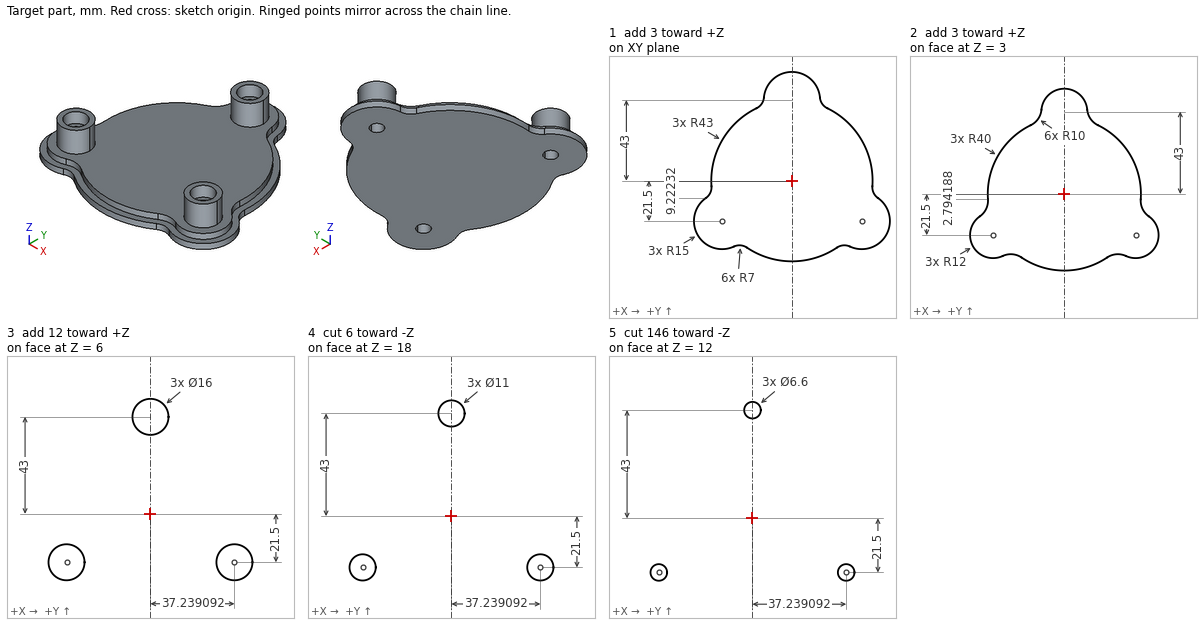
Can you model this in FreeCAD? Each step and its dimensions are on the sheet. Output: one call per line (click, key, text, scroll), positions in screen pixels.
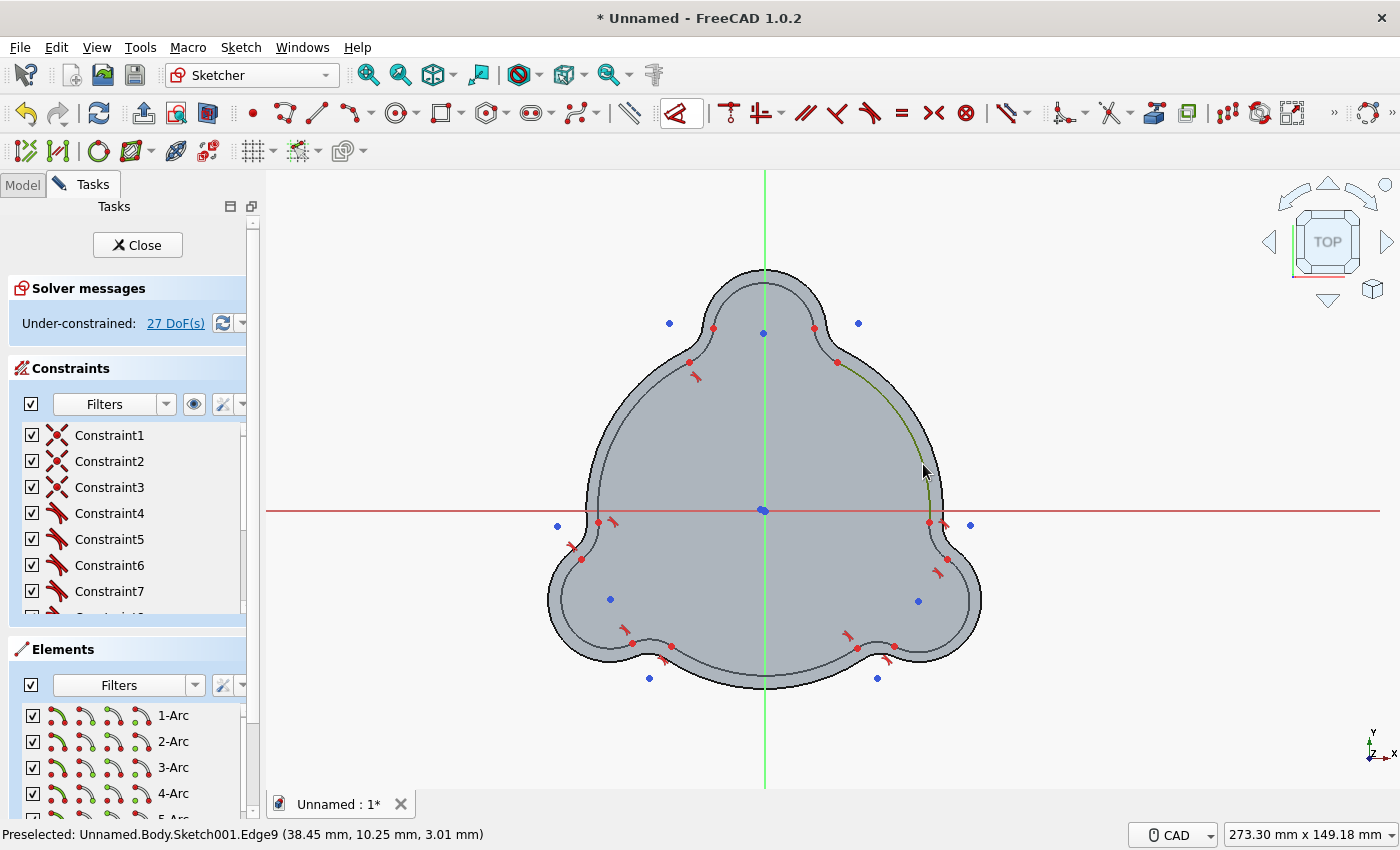
click(817, 341)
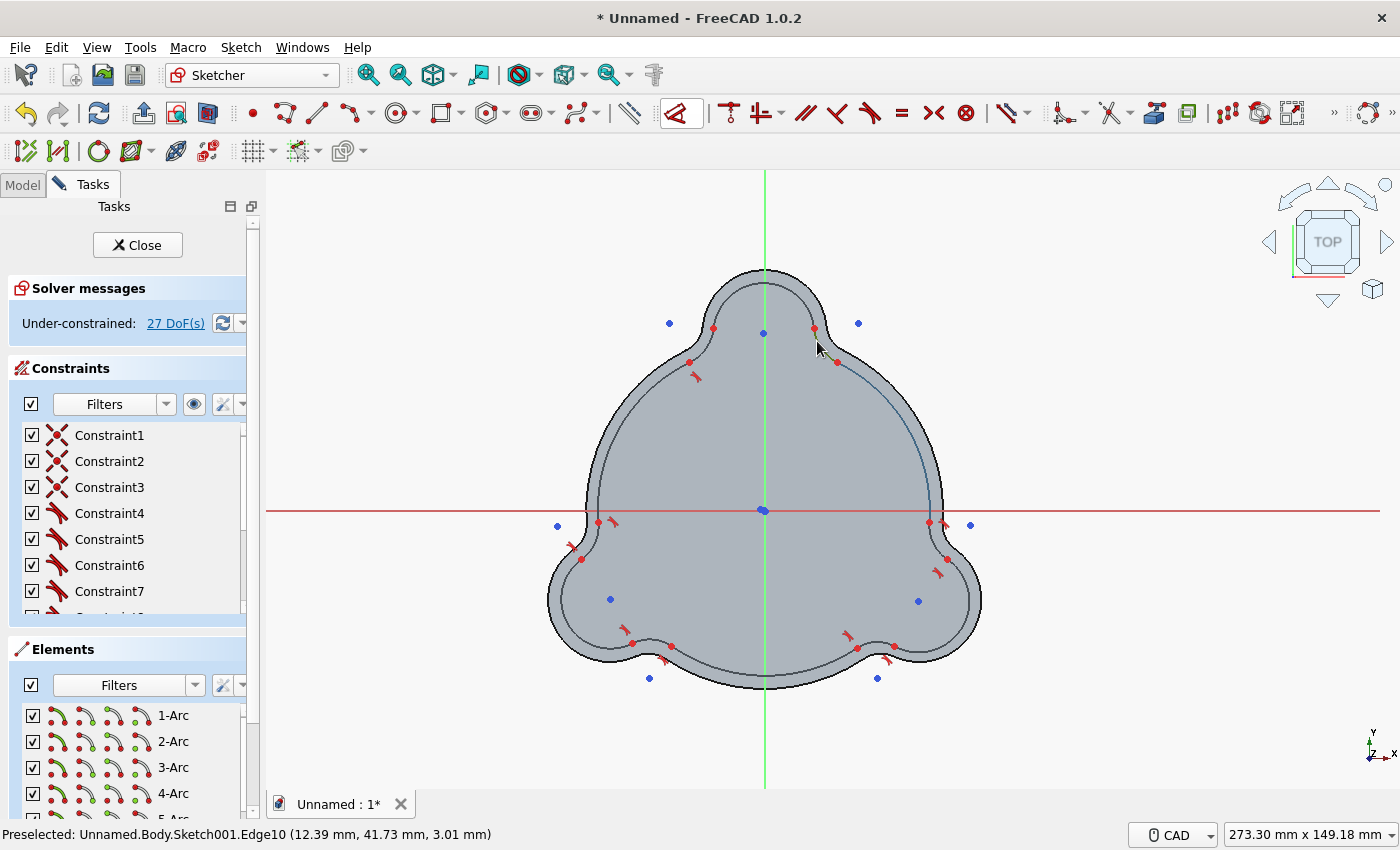
click(870, 114)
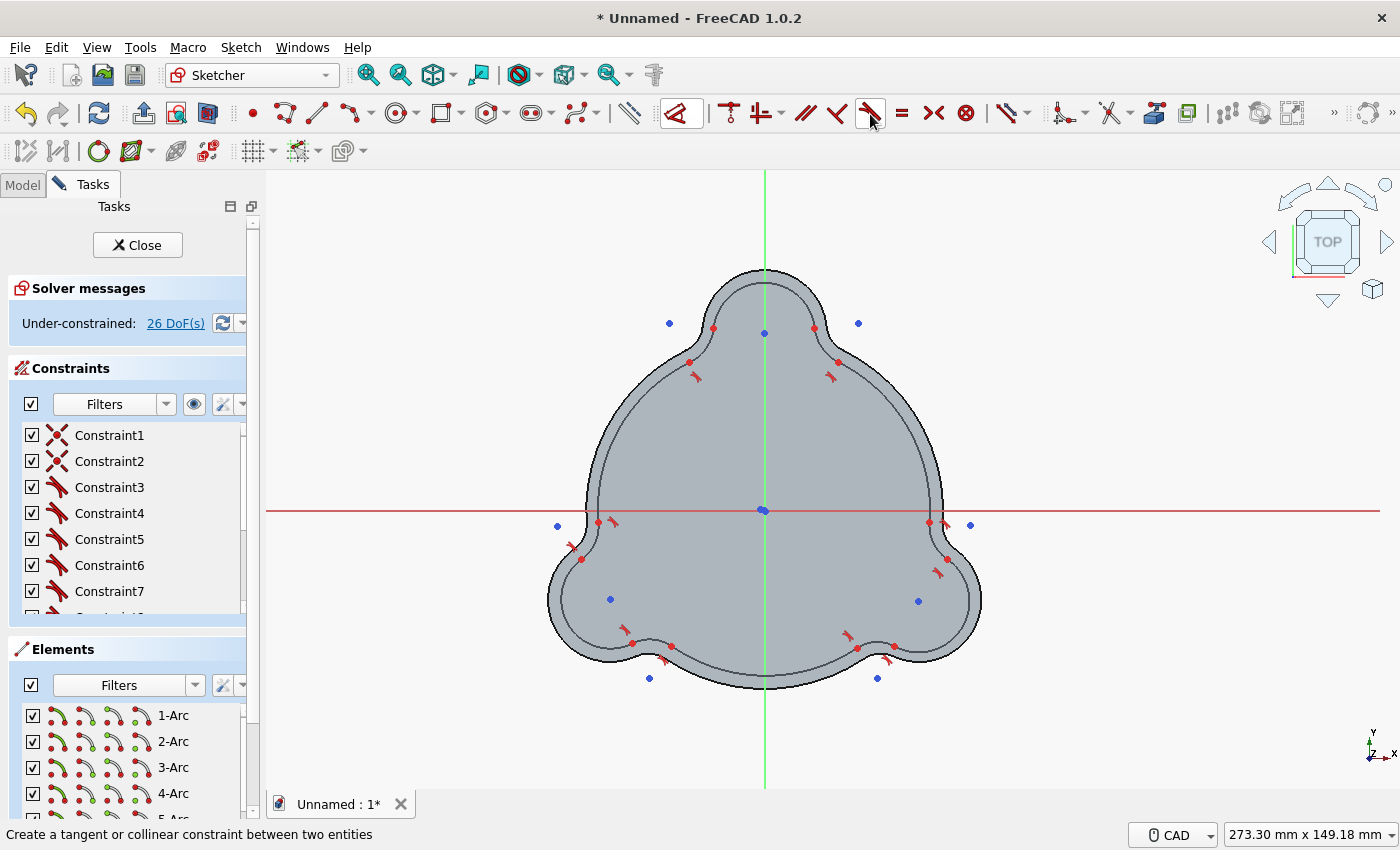
click(818, 341)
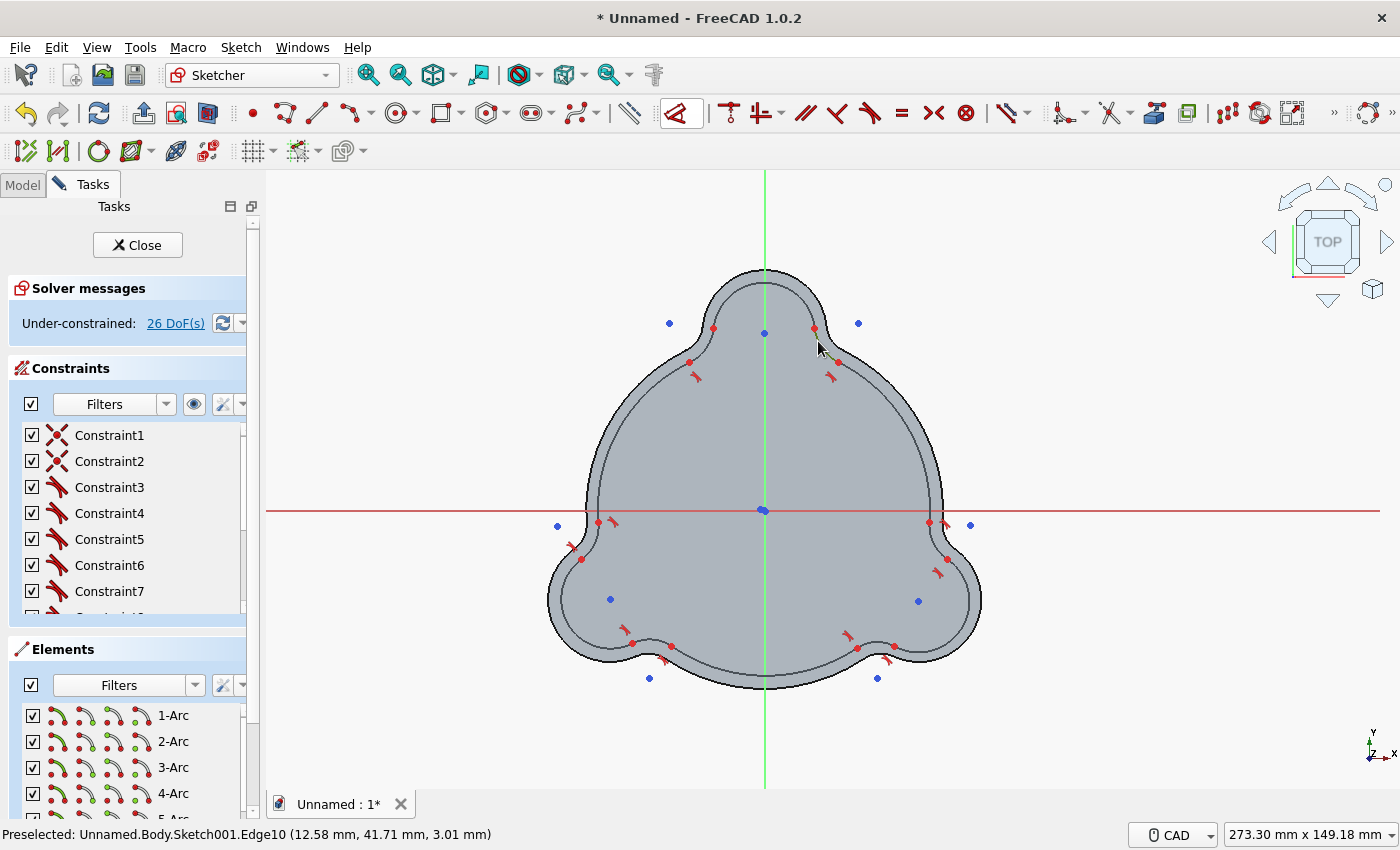
click(792, 291)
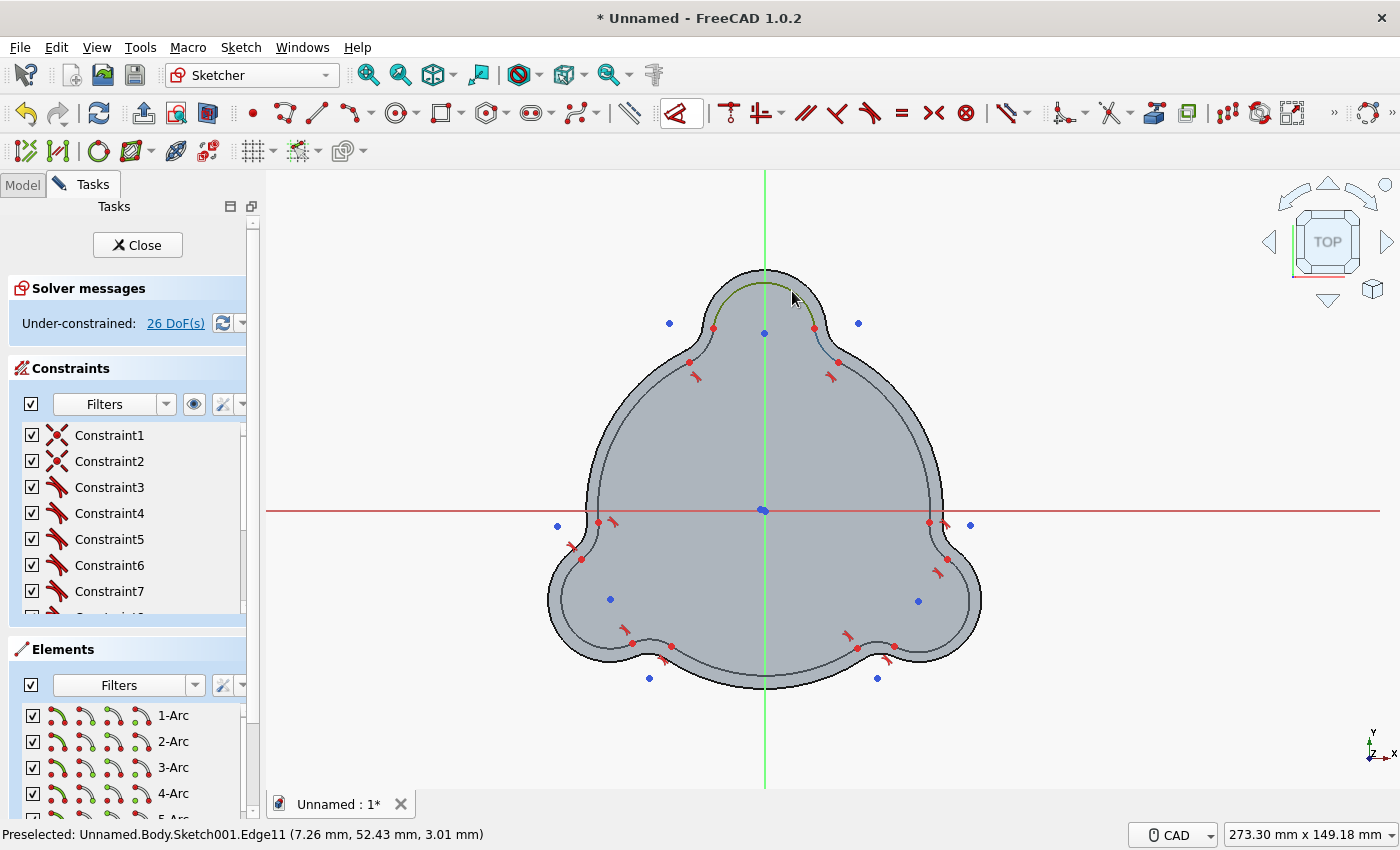
click(870, 114)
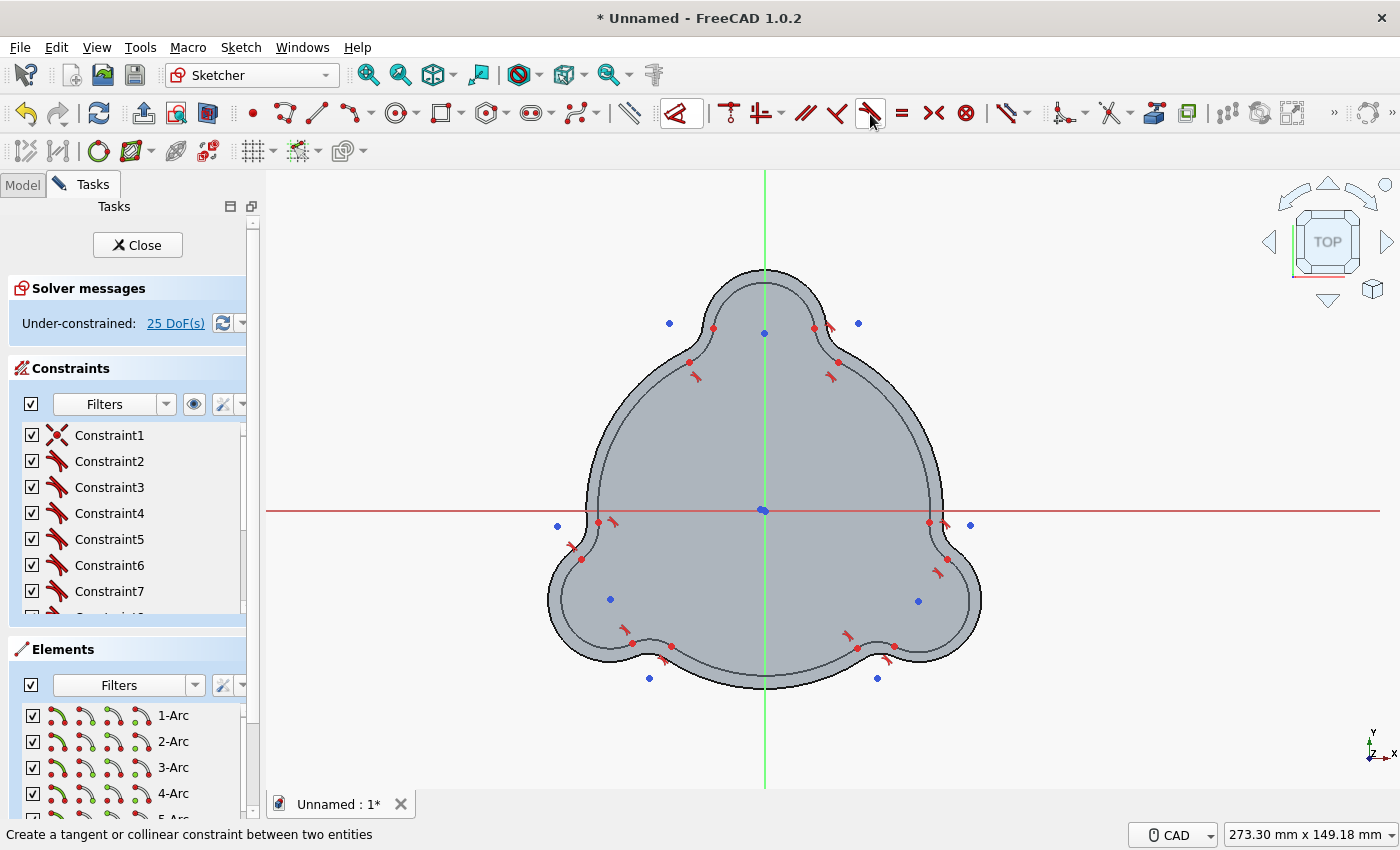
click(792, 291)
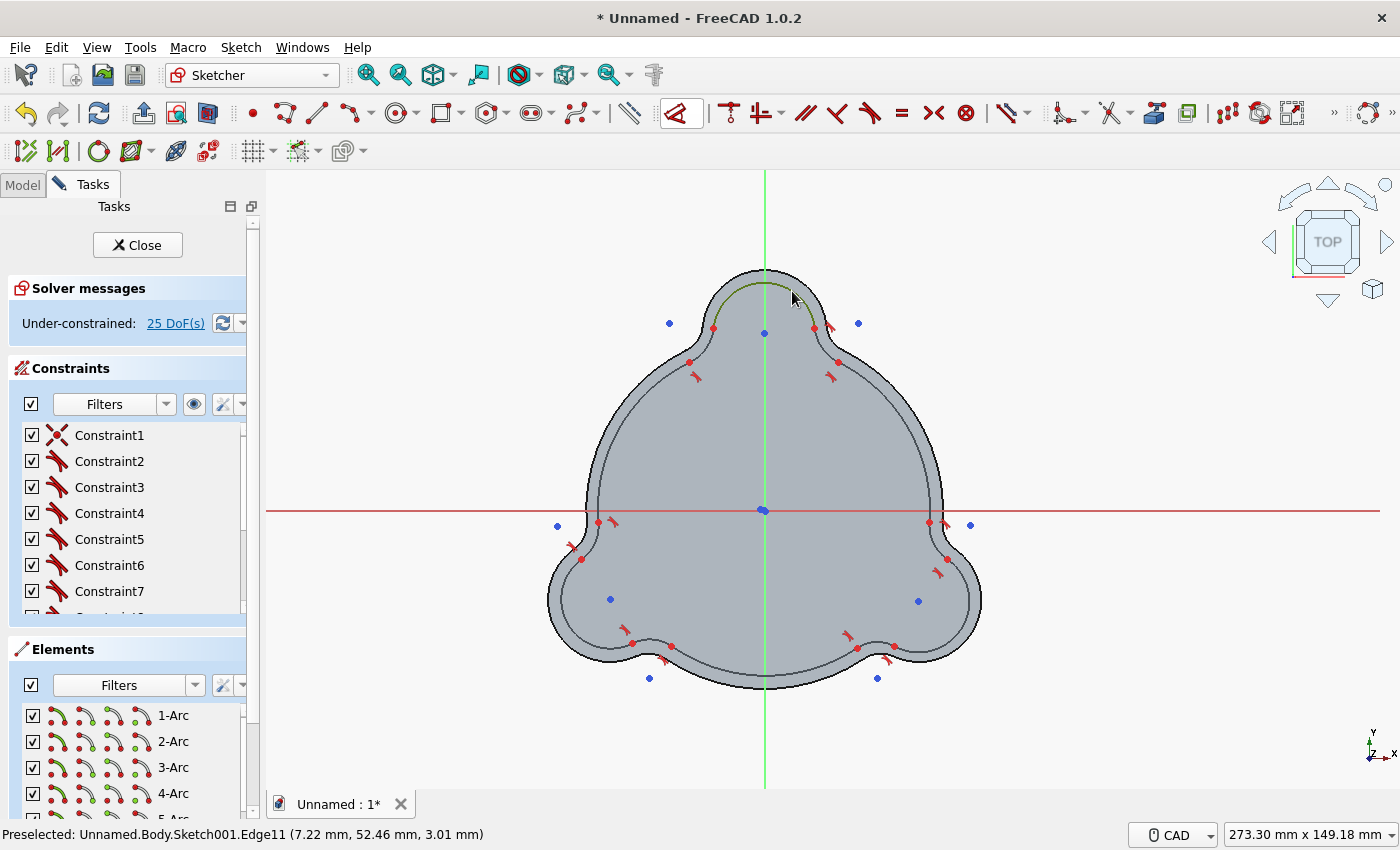
click(700, 355)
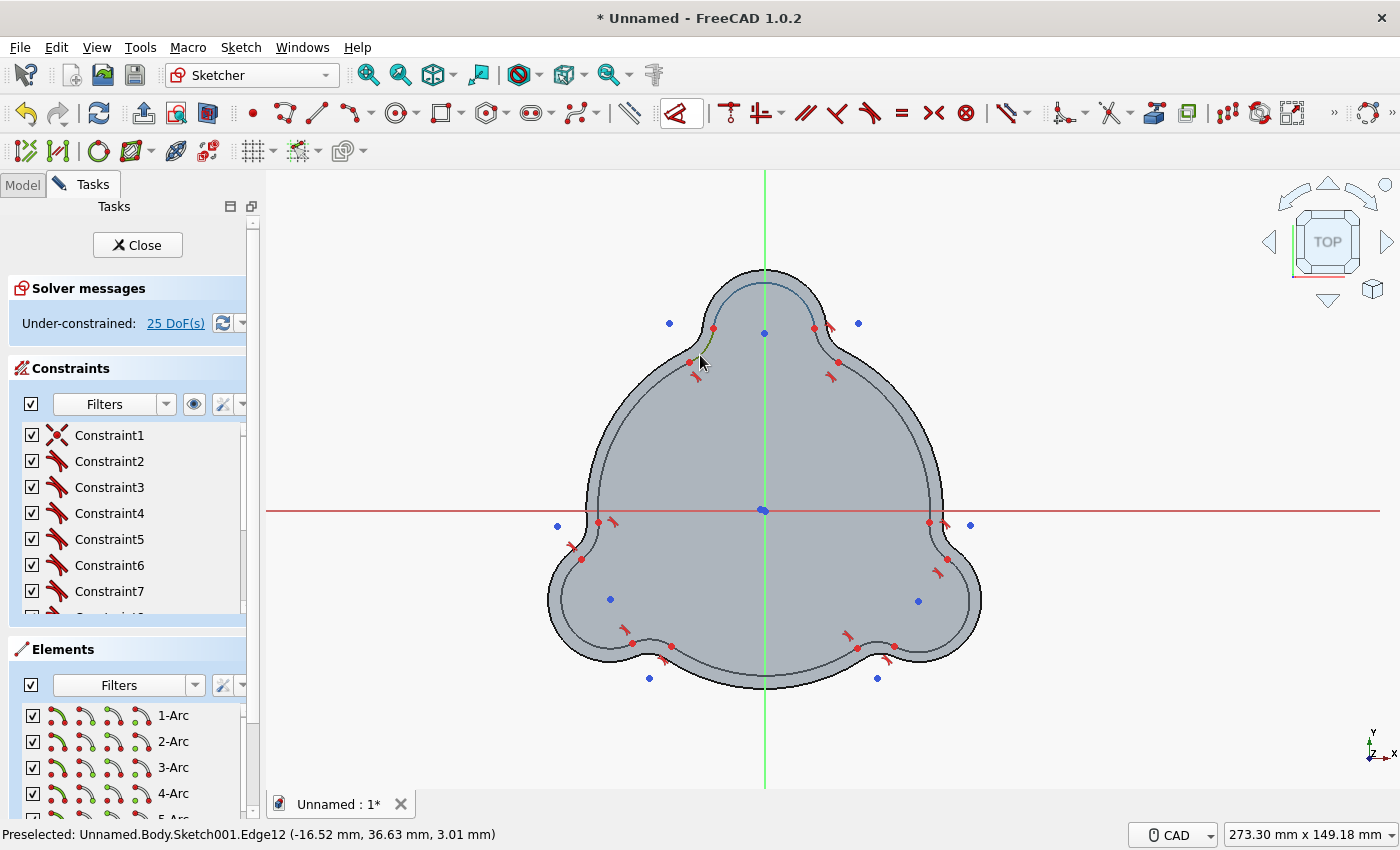
click(870, 114)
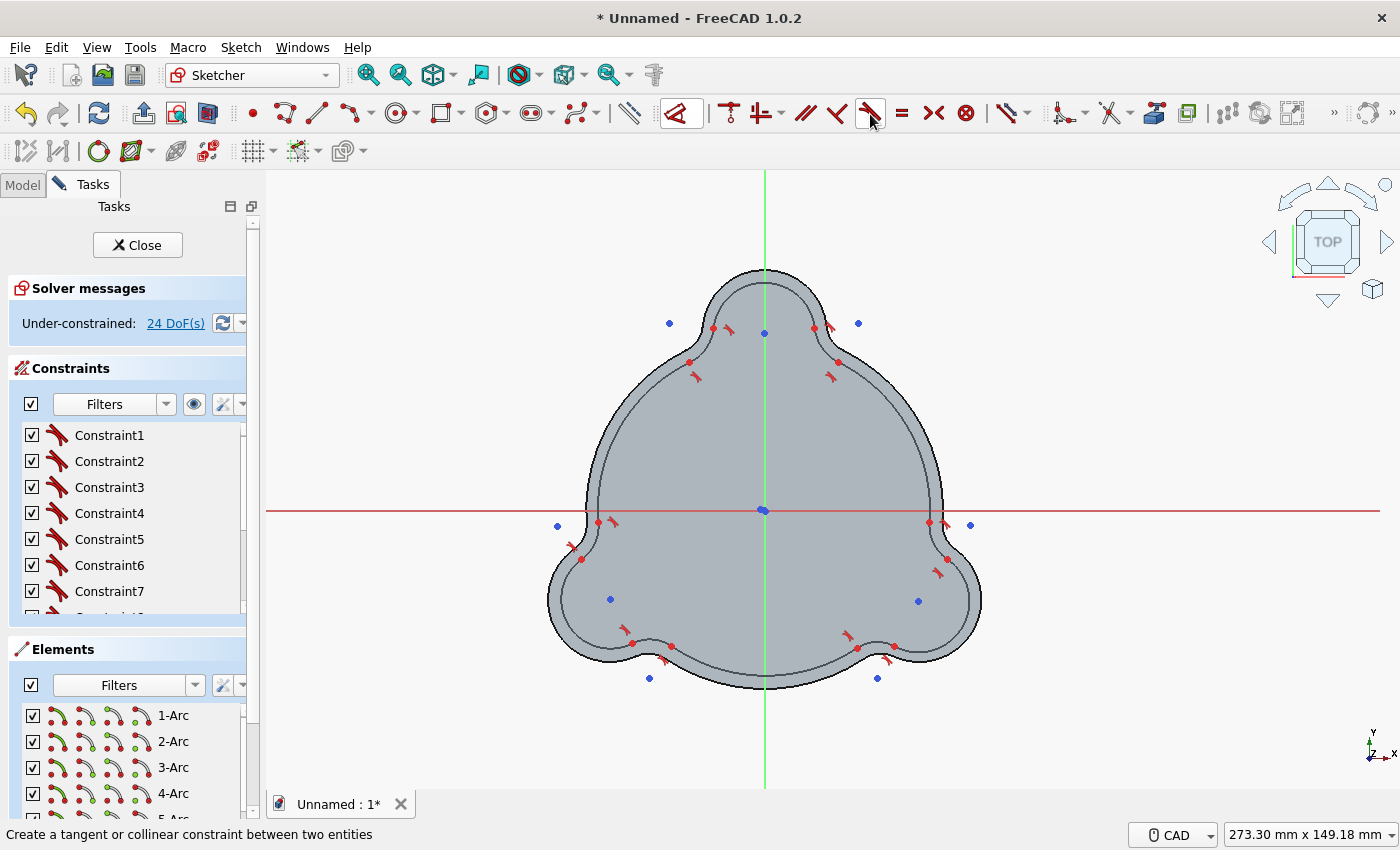
click(642, 397)